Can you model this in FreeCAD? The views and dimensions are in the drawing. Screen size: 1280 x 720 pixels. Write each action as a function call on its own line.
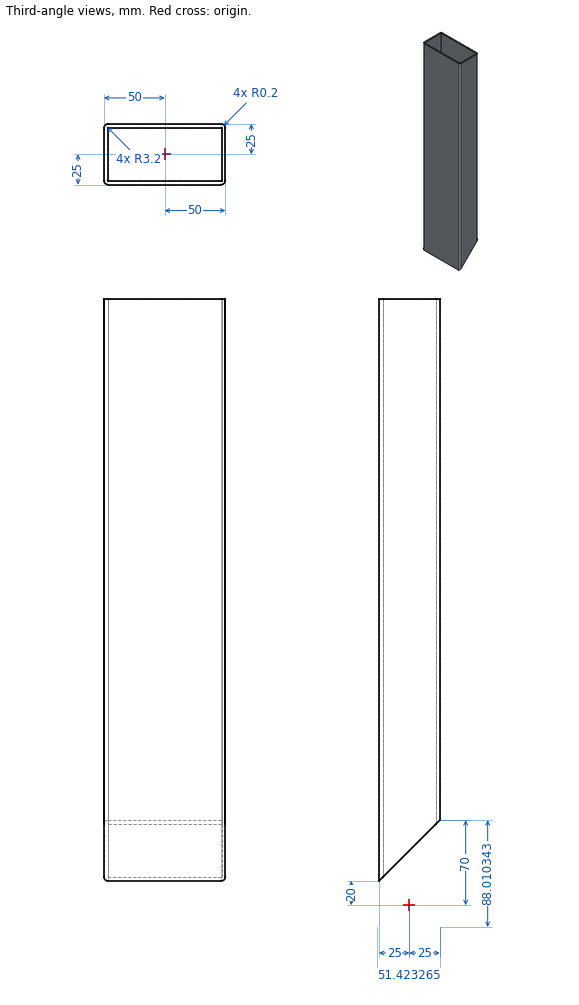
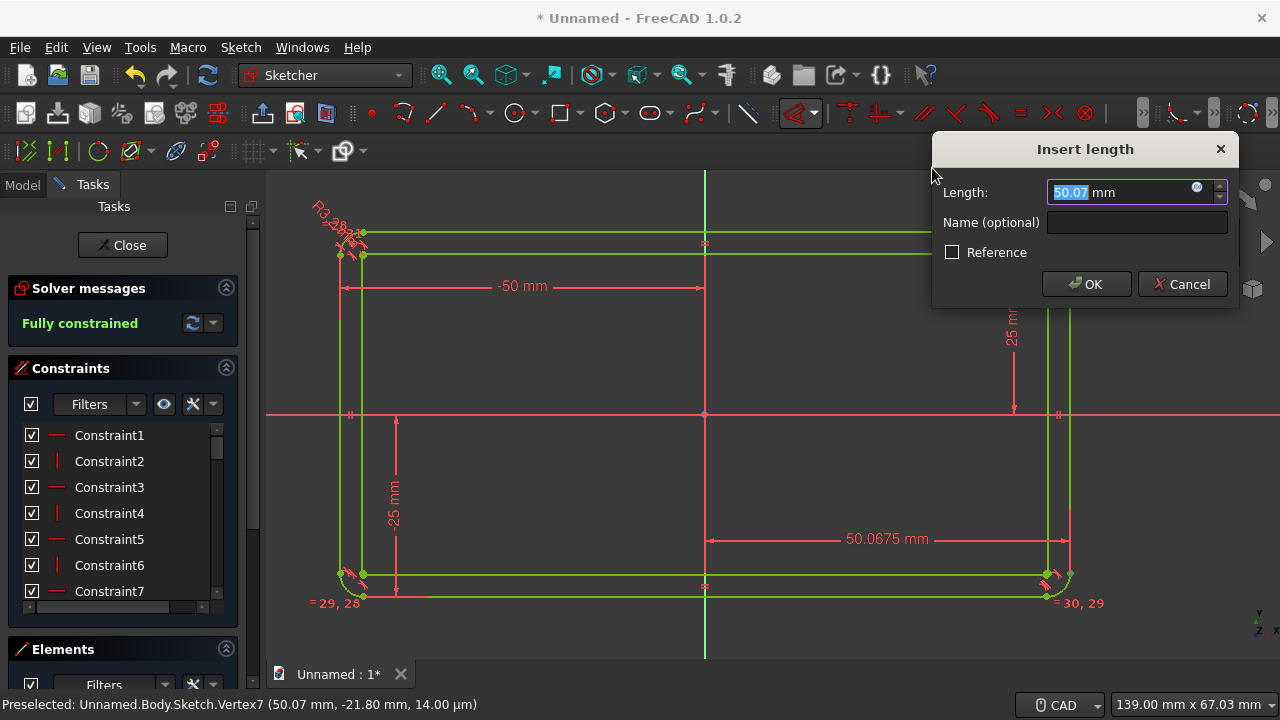
text(50)
key(Return)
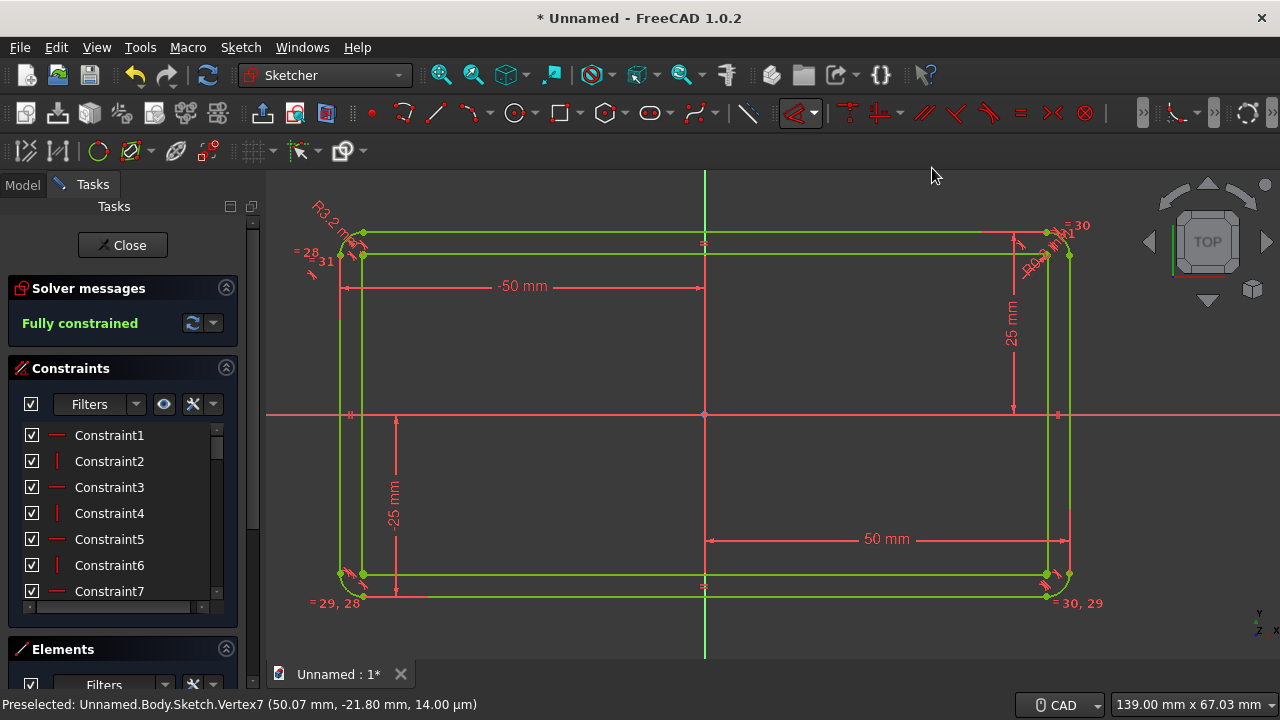
click(123, 245)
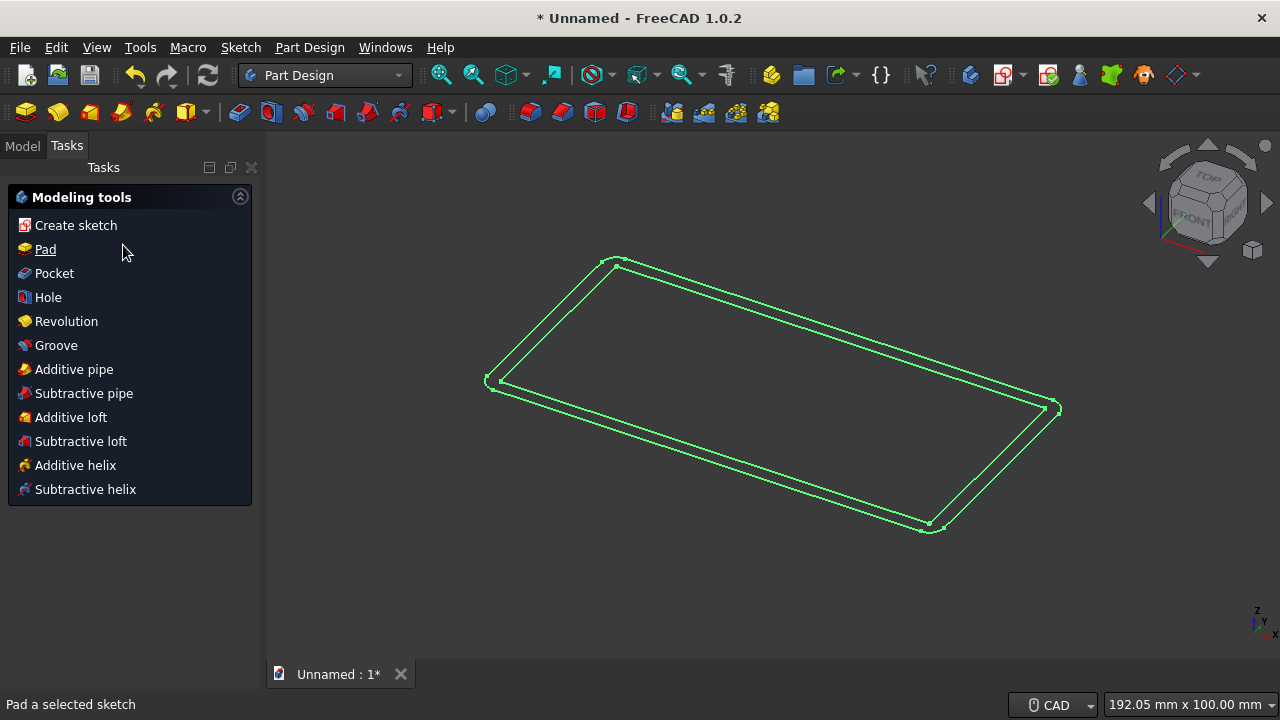
click(26, 112)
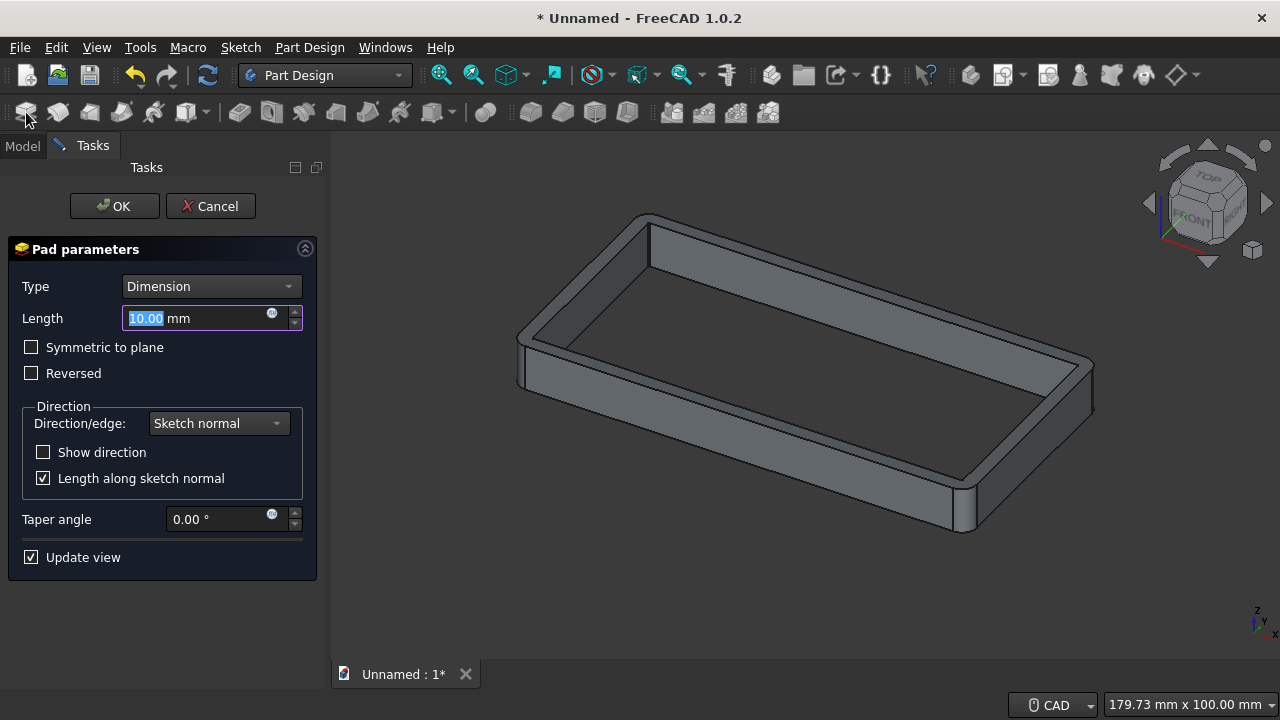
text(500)
key(Tab)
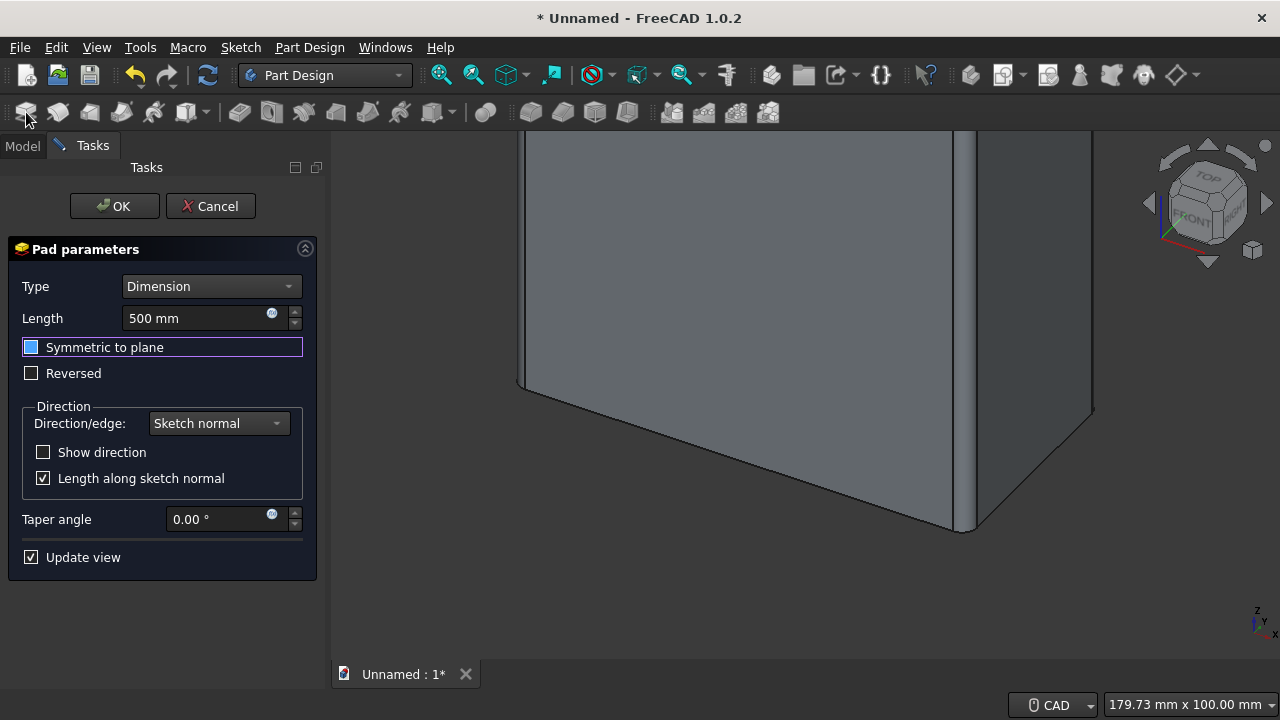
click(115, 206)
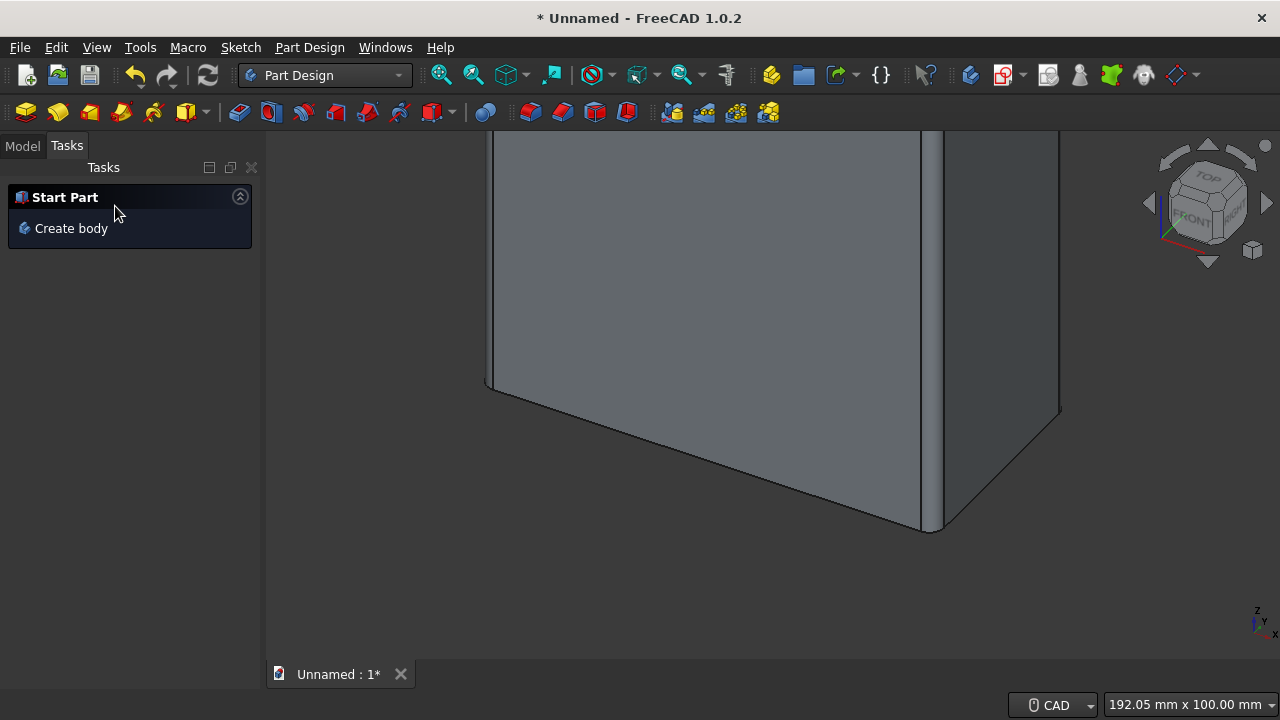
click(442, 76)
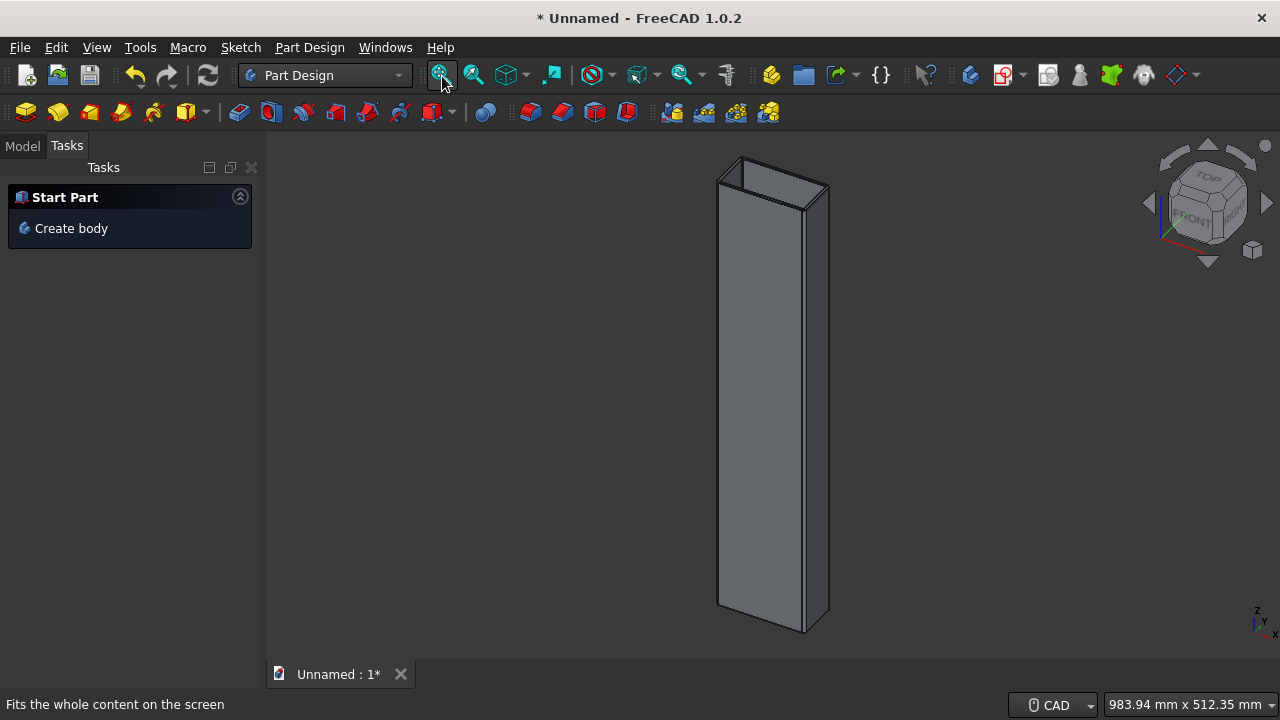
click(818, 228)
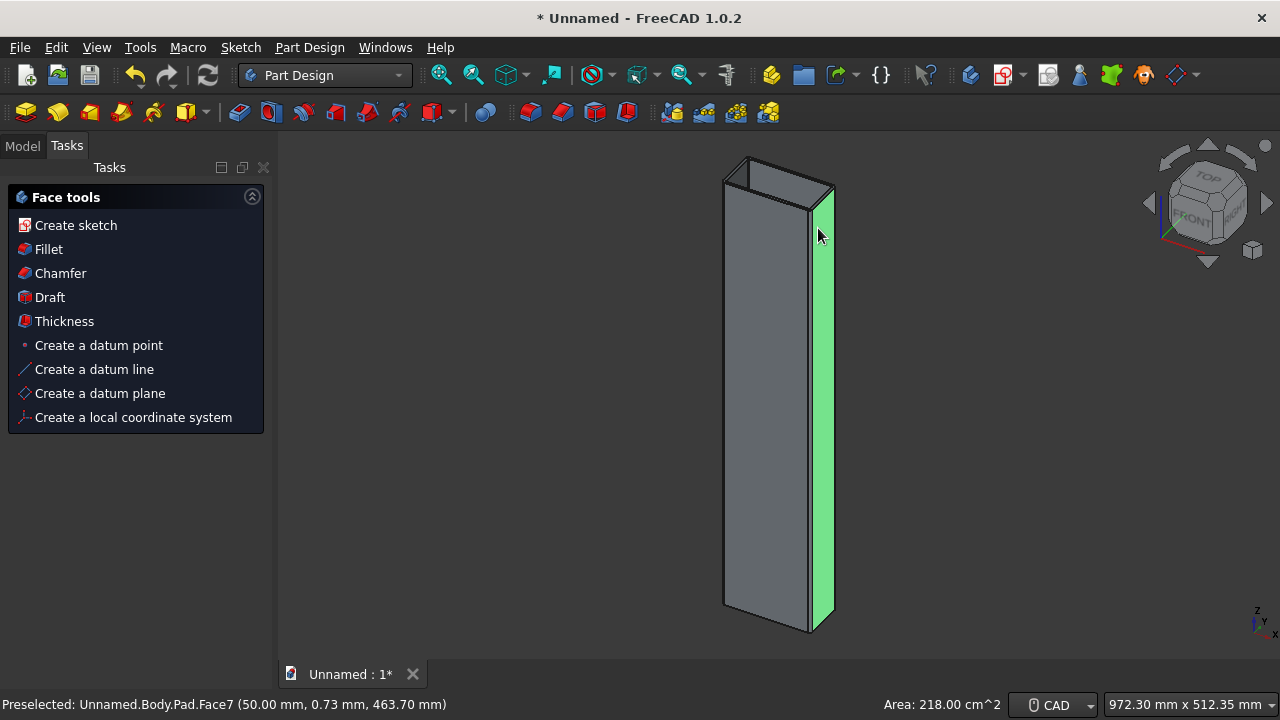
click(1004, 76)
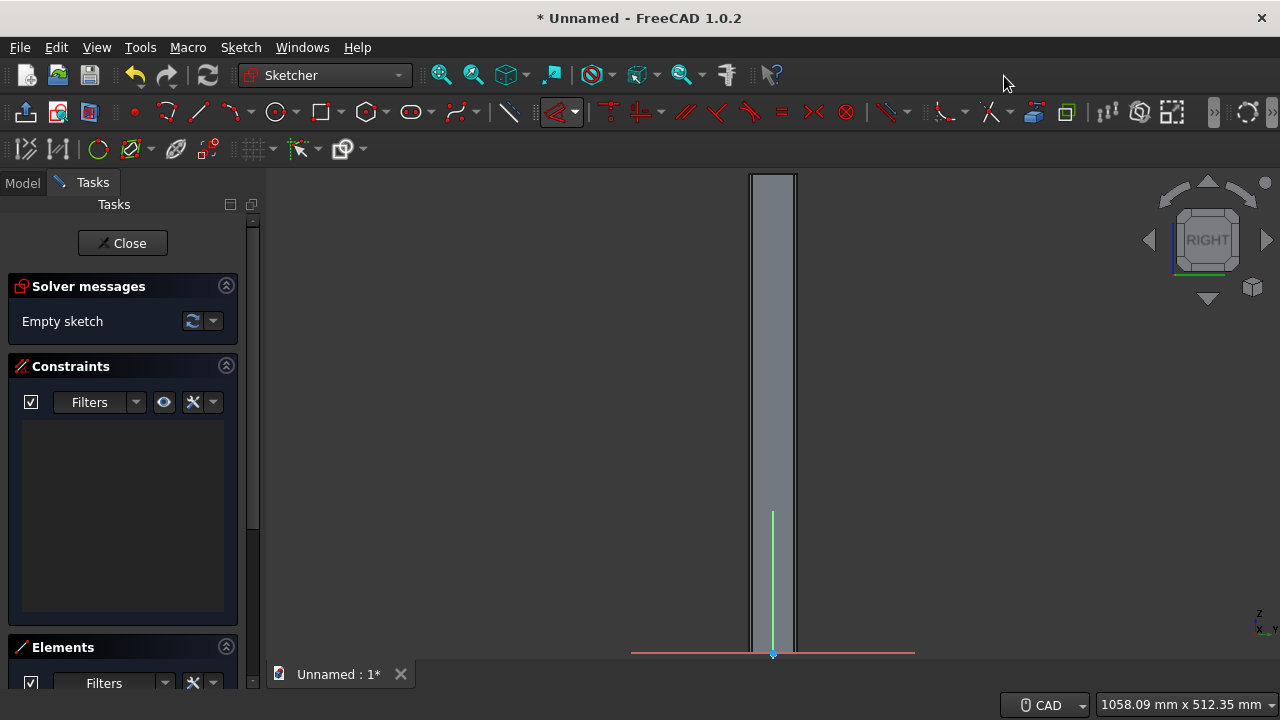
scroll(704, 414, down, 5)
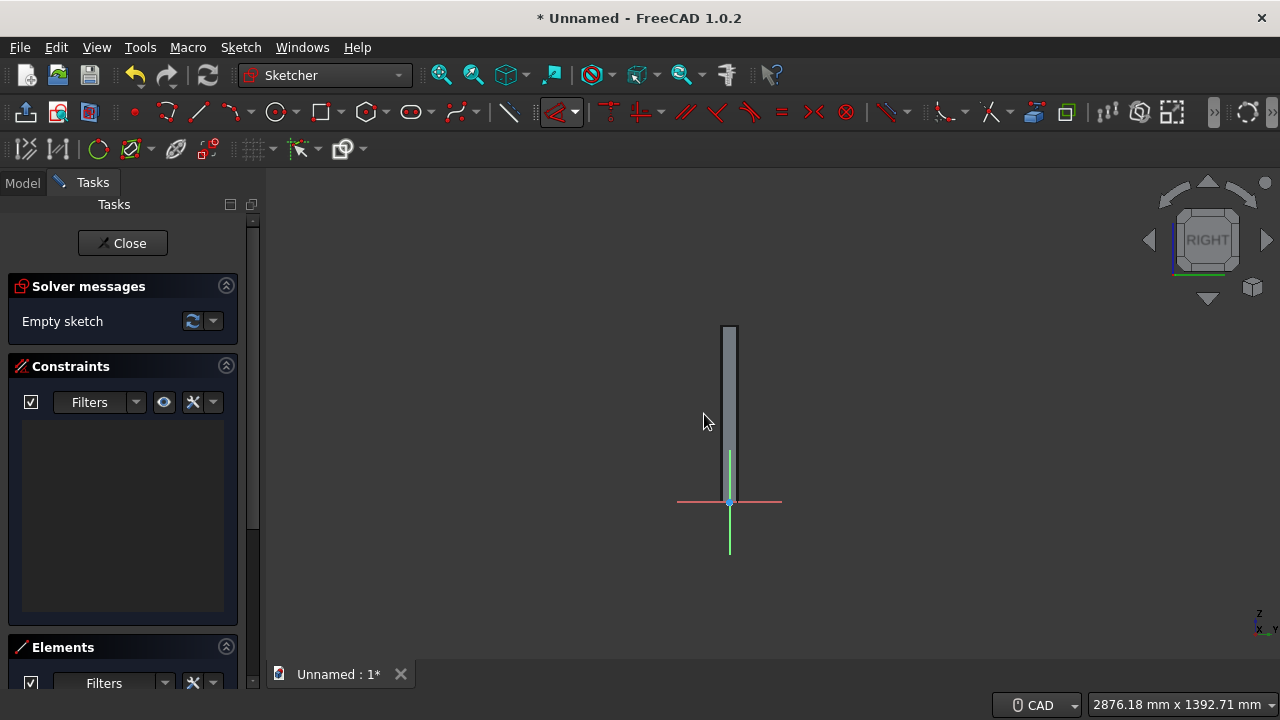
scroll(733, 503, up, 11)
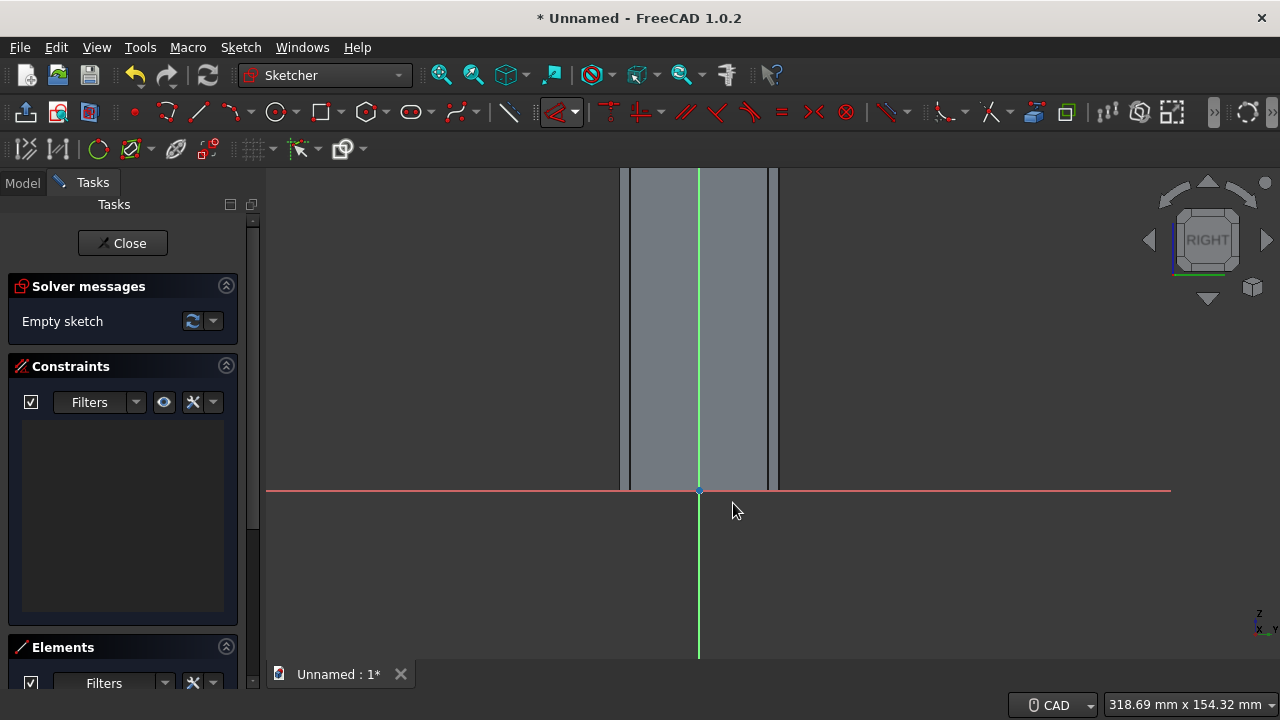
click(168, 112)